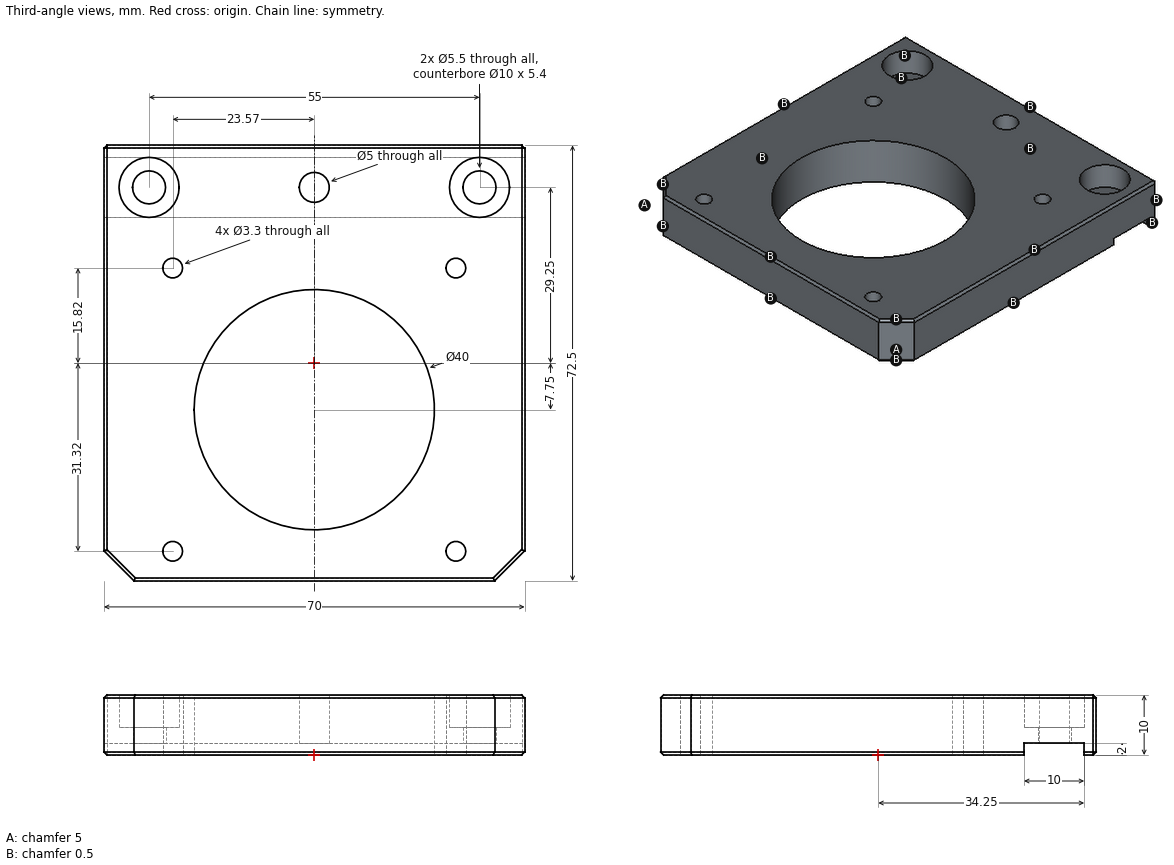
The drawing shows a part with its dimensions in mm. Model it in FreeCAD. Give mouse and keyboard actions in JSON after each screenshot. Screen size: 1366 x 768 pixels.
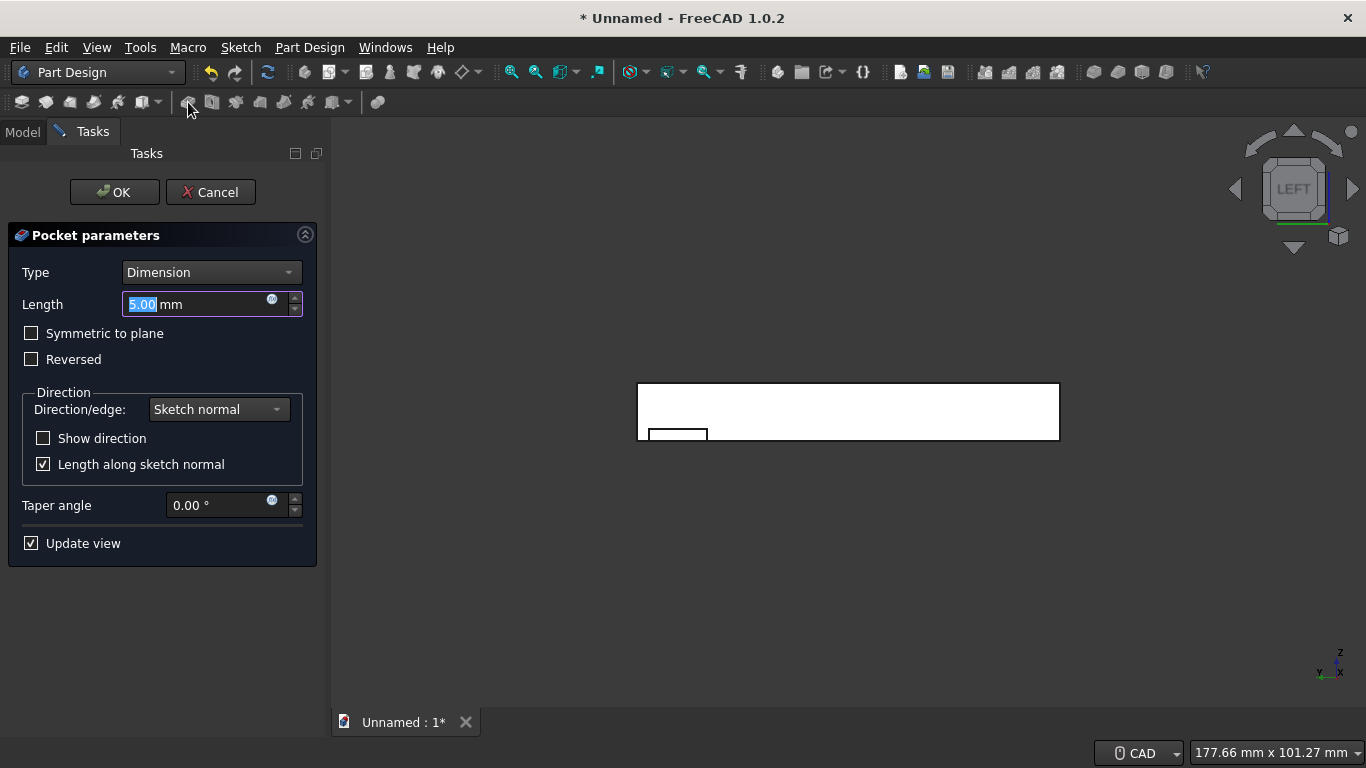
{"action": "left_click", "coordinate": [212, 272]}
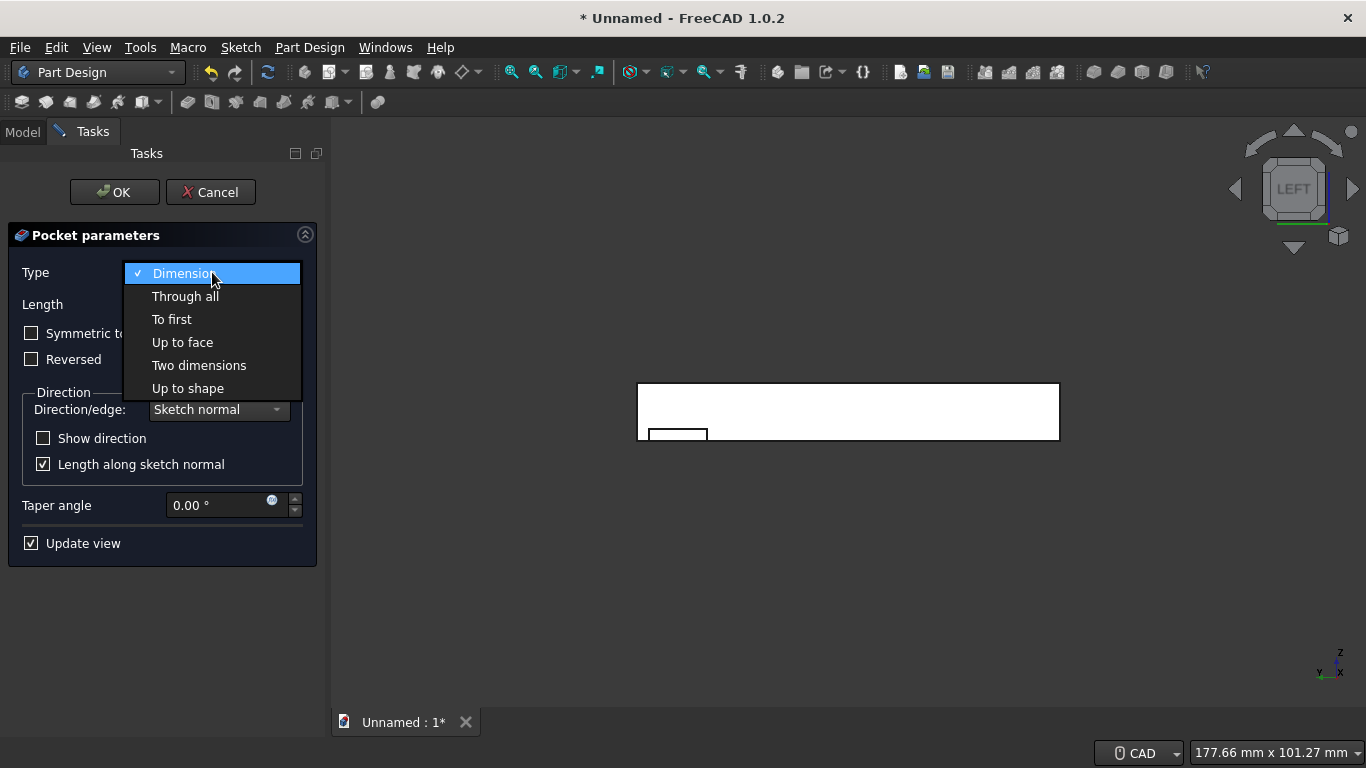
{"action": "left_click", "coordinate": [212, 296]}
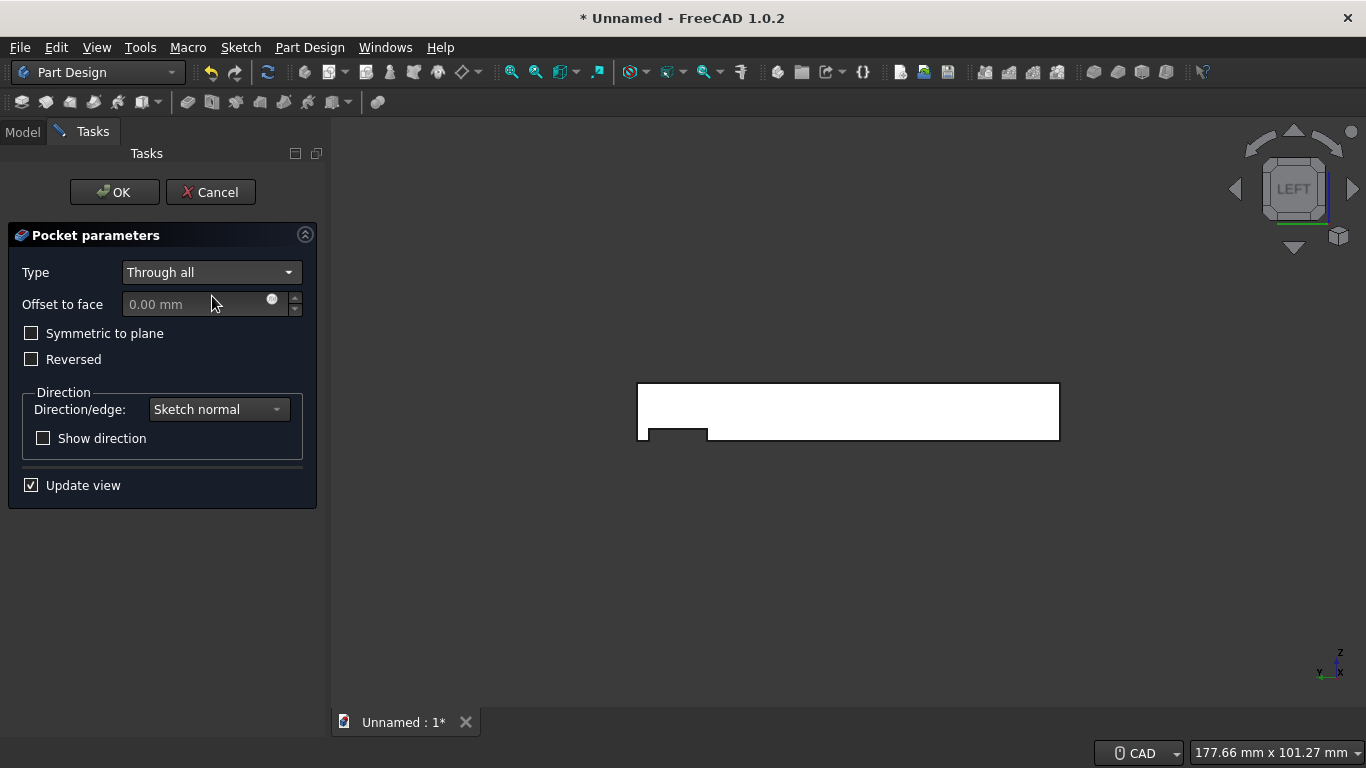
{"action": "left_click", "coordinate": [115, 192]}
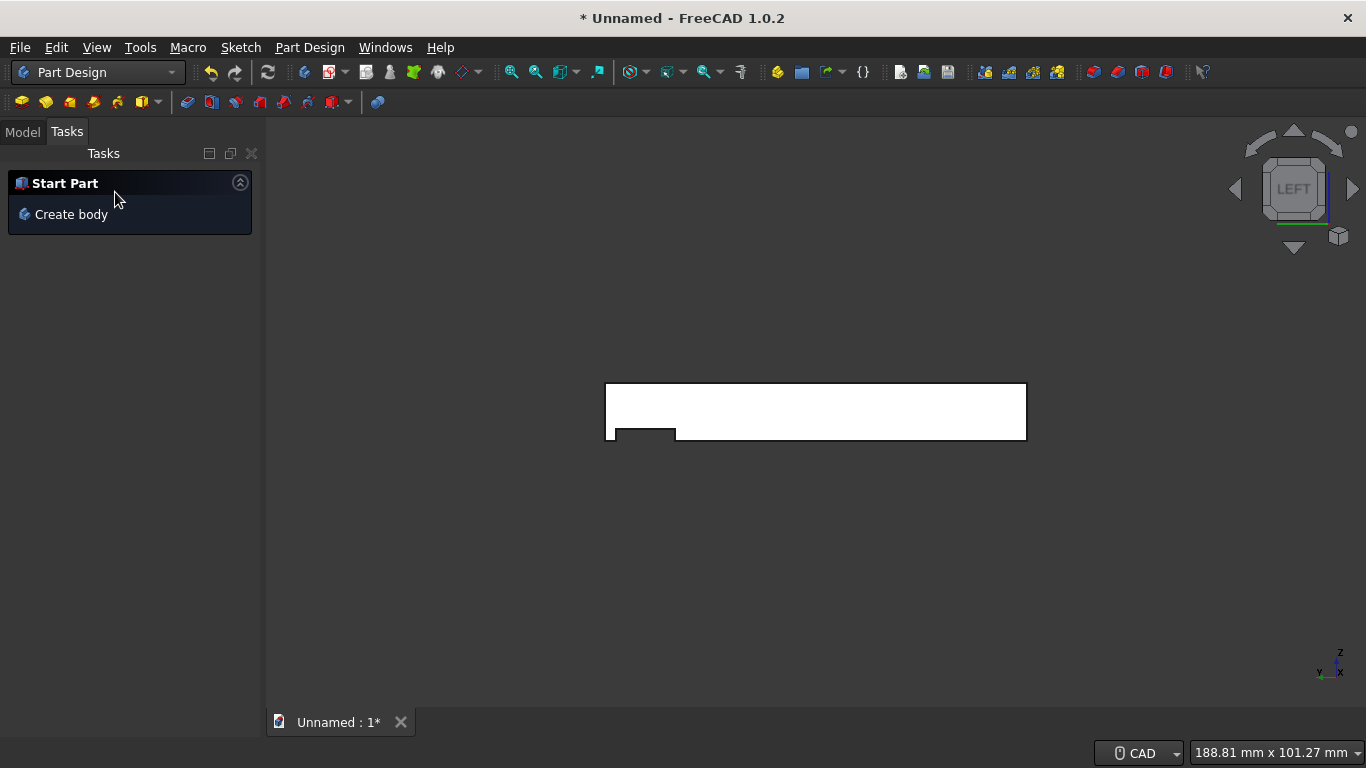
{"action": "left_click", "coordinate": [512, 72]}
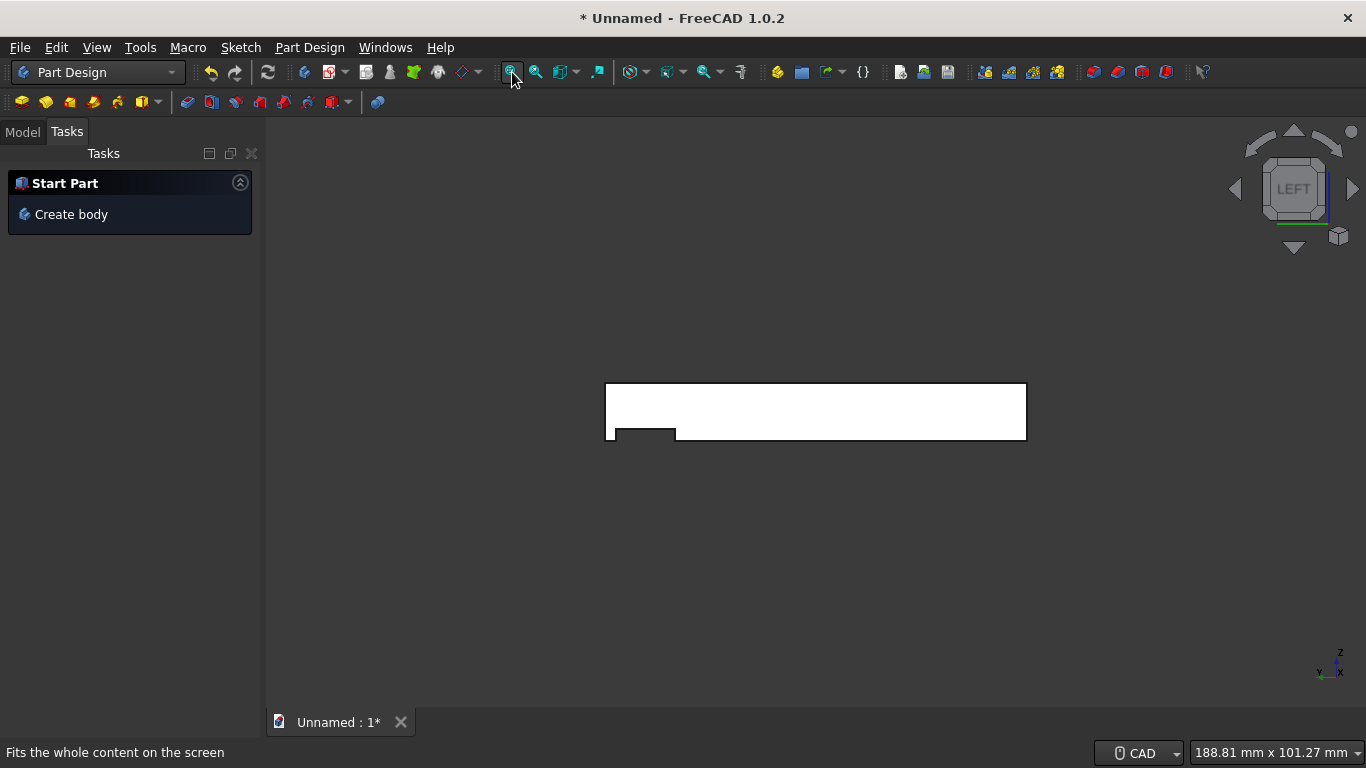
{"action": "key", "text": "0"}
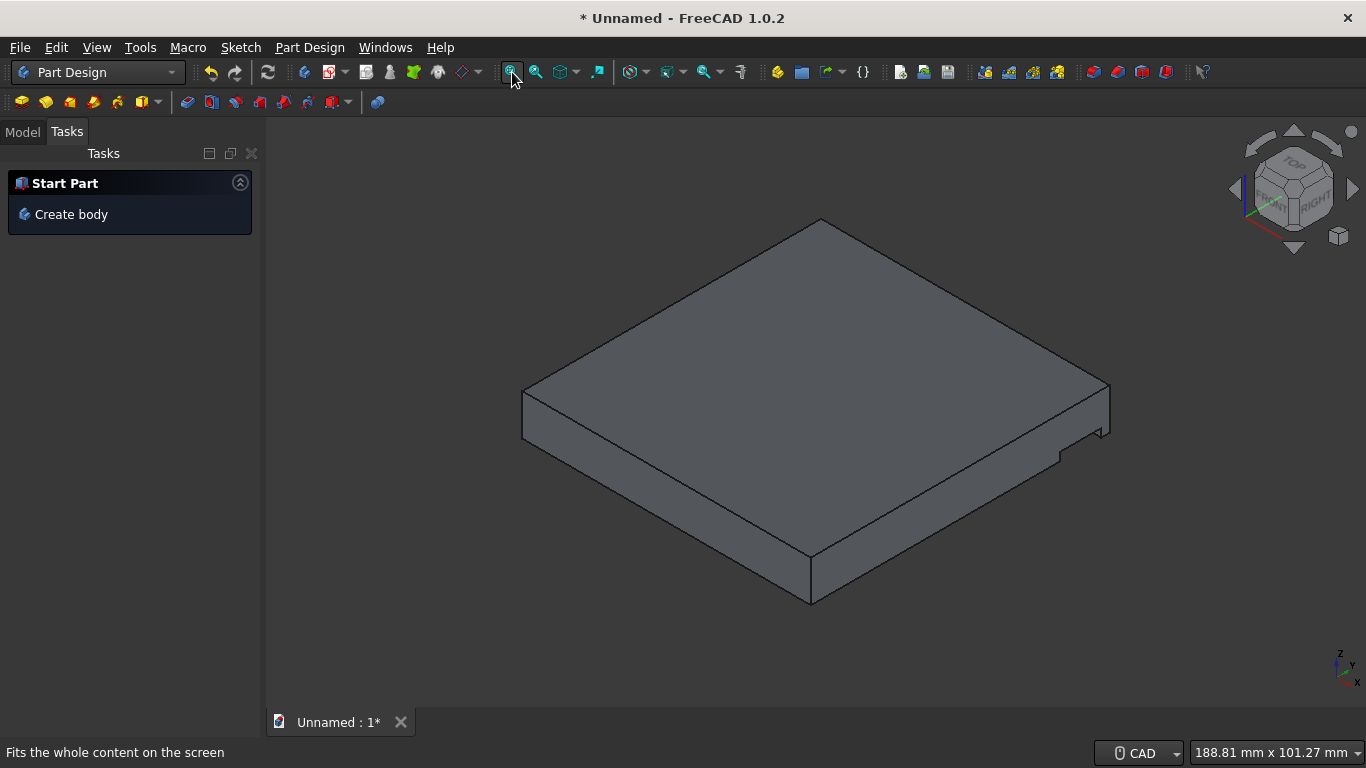
{"action": "left_click", "coordinate": [816, 387]}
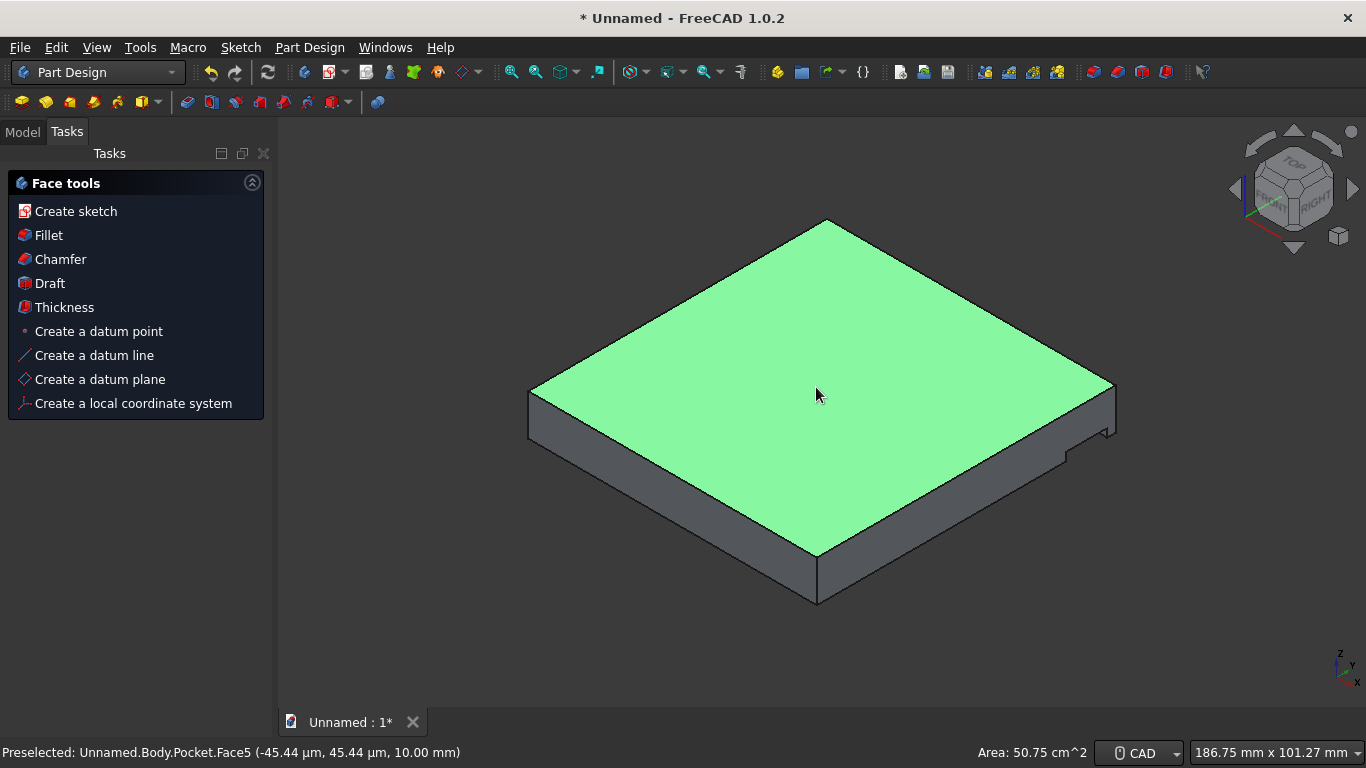
{"action": "left_click", "coordinate": [330, 72]}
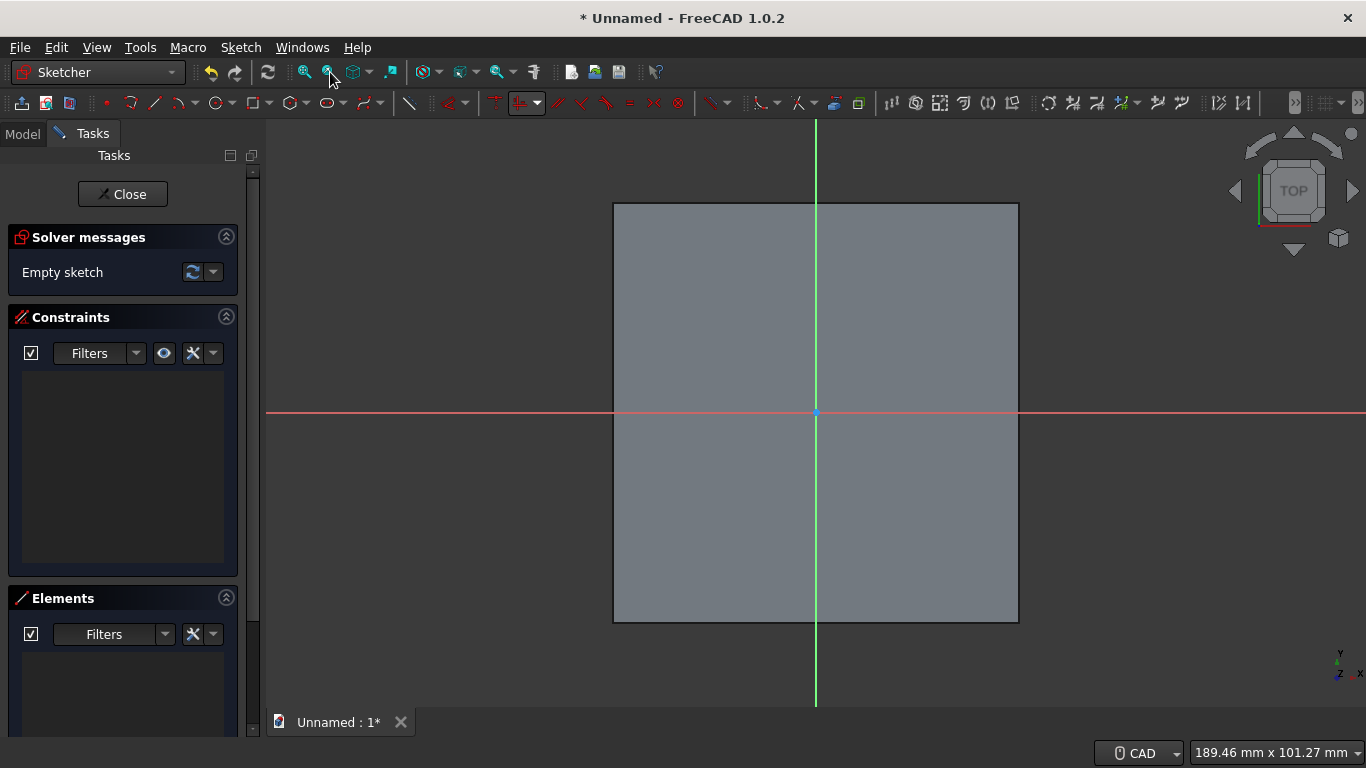
{"action": "scroll", "coordinate": [899, 207], "scroll_direction": "up", "scroll_amount": 3}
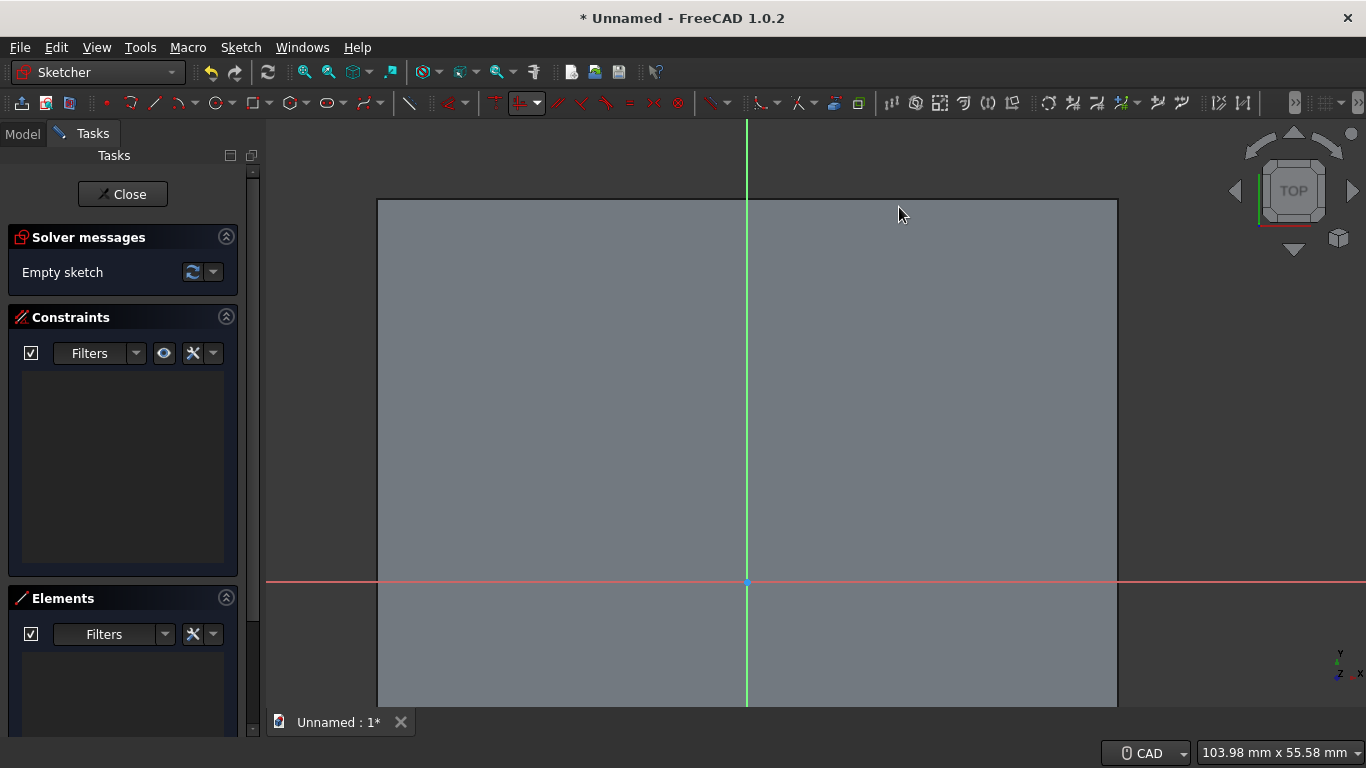
{"action": "left_click", "coordinate": [216, 104]}